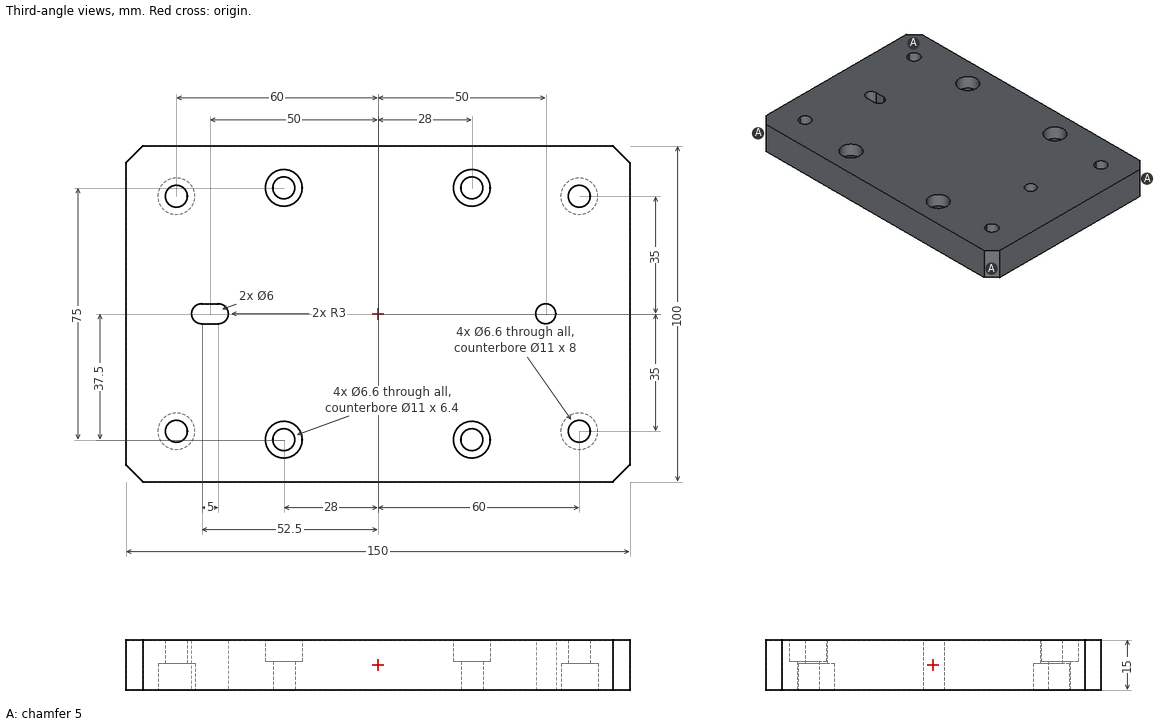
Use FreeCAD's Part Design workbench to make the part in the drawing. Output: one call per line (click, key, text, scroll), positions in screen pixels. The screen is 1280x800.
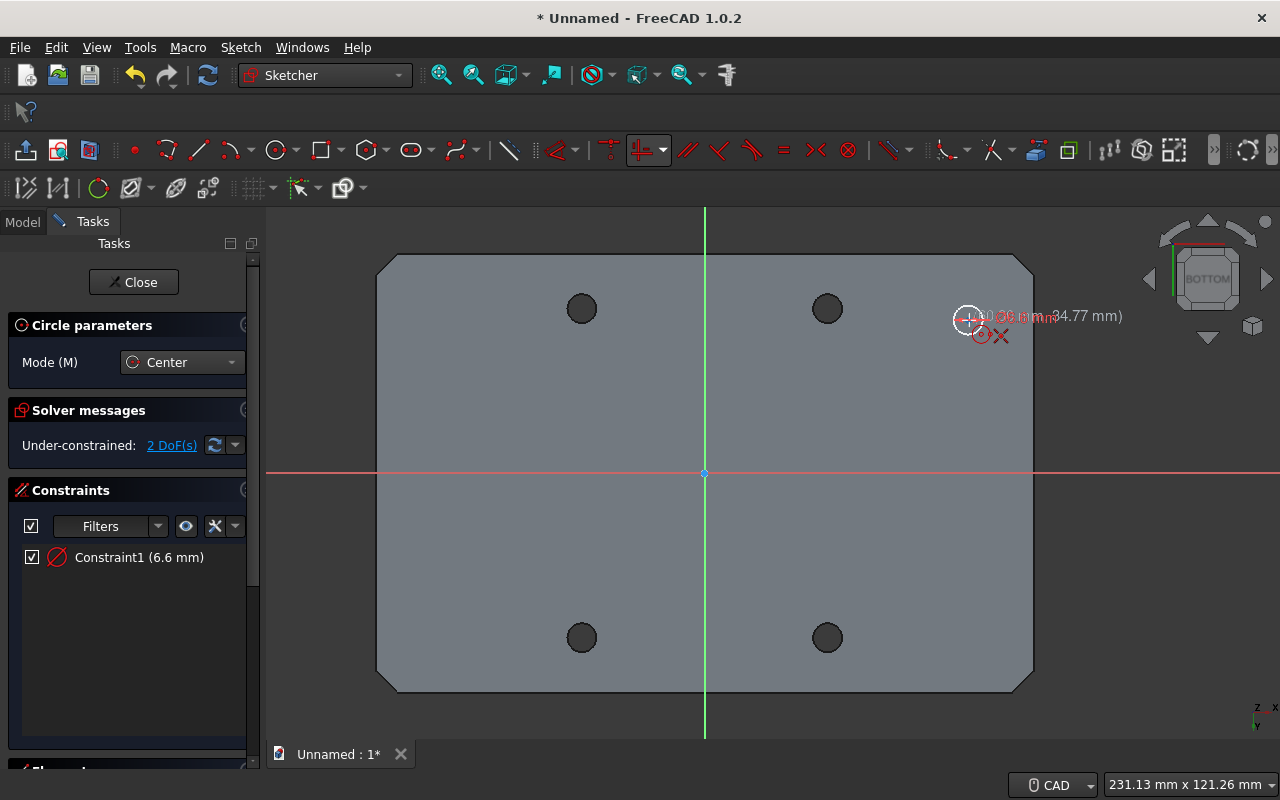
scroll(968, 627, up, 3)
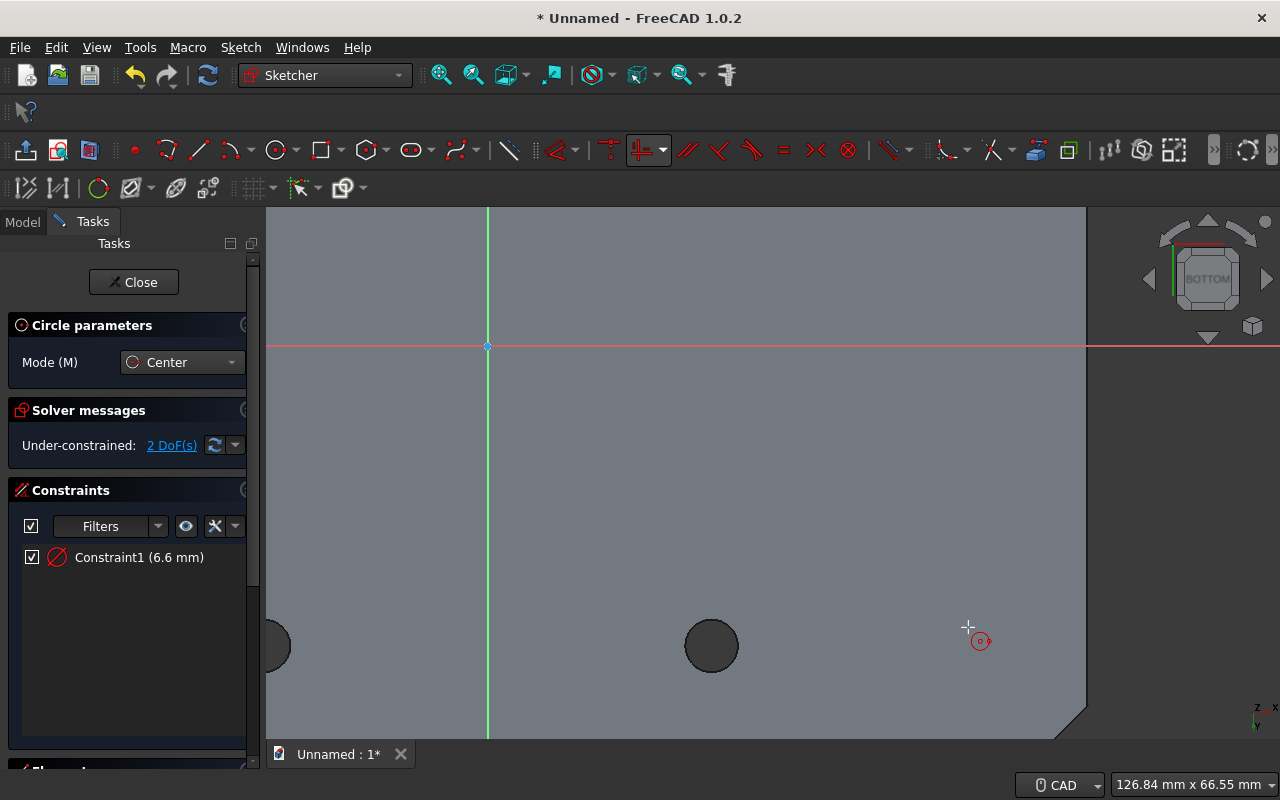
click(967, 626)
move(986, 607)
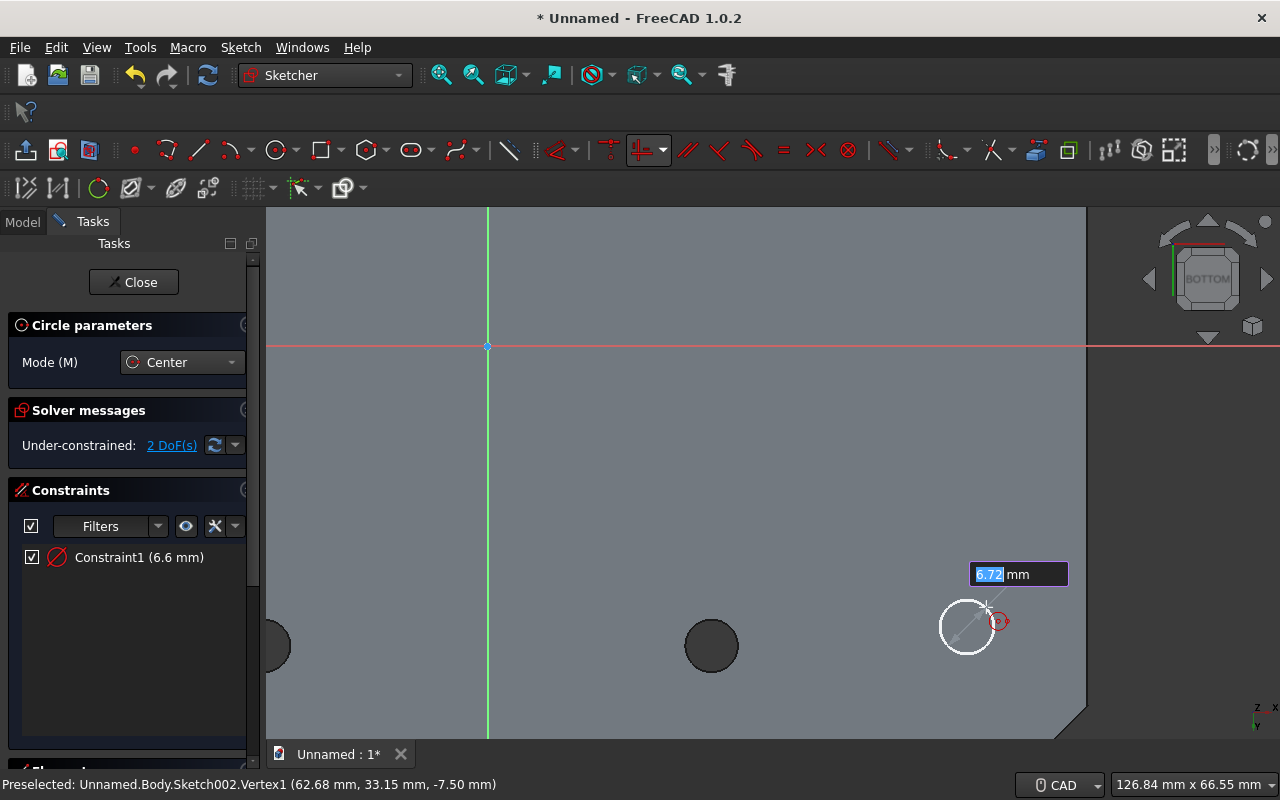
text(6.6)
key(Return)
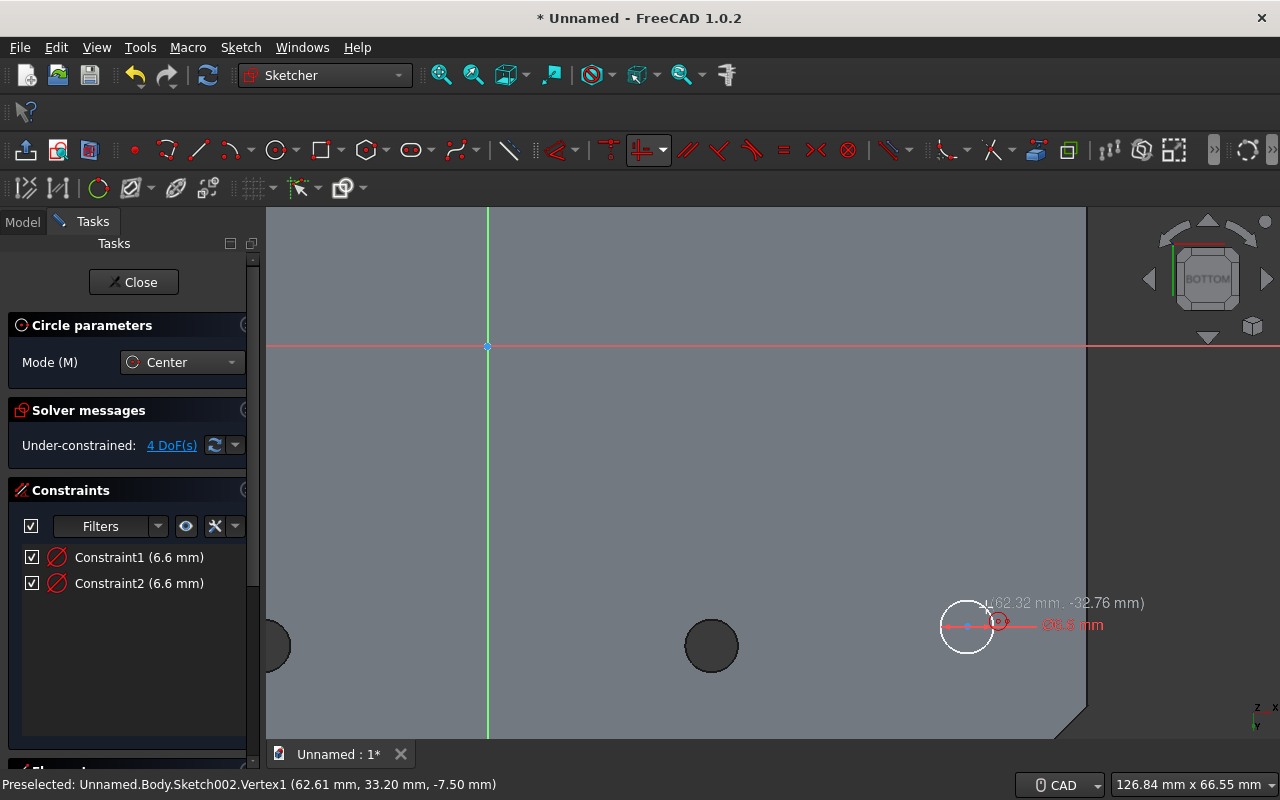
scroll(968, 627, down, 3)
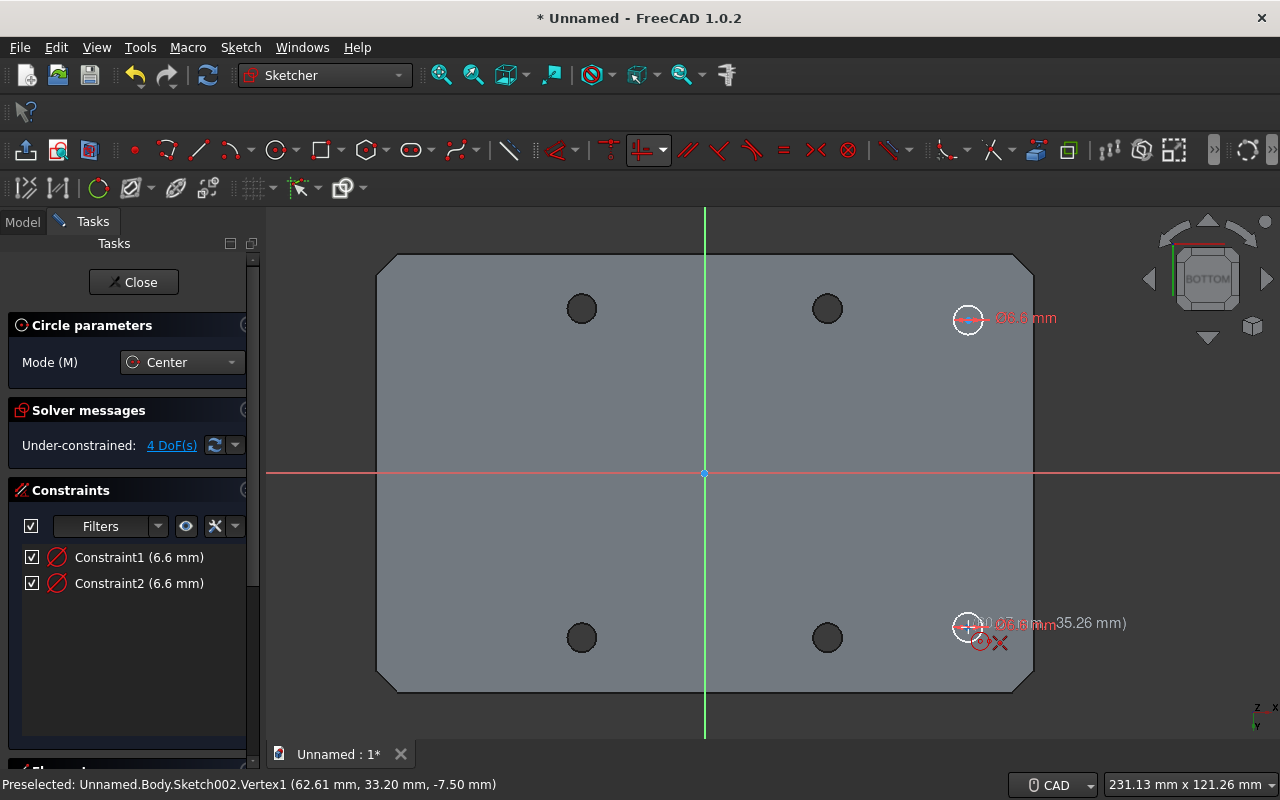
scroll(442, 627, up, 3)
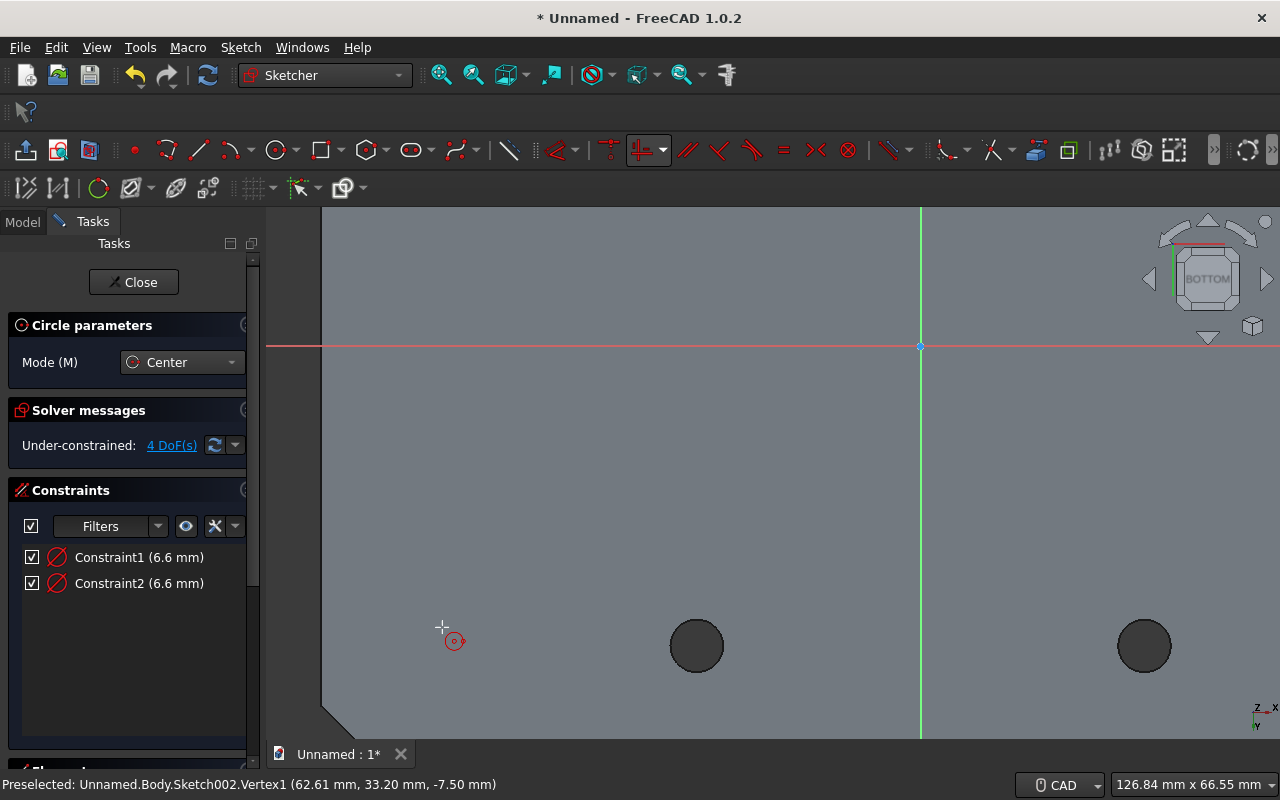
click(441, 626)
move(460, 607)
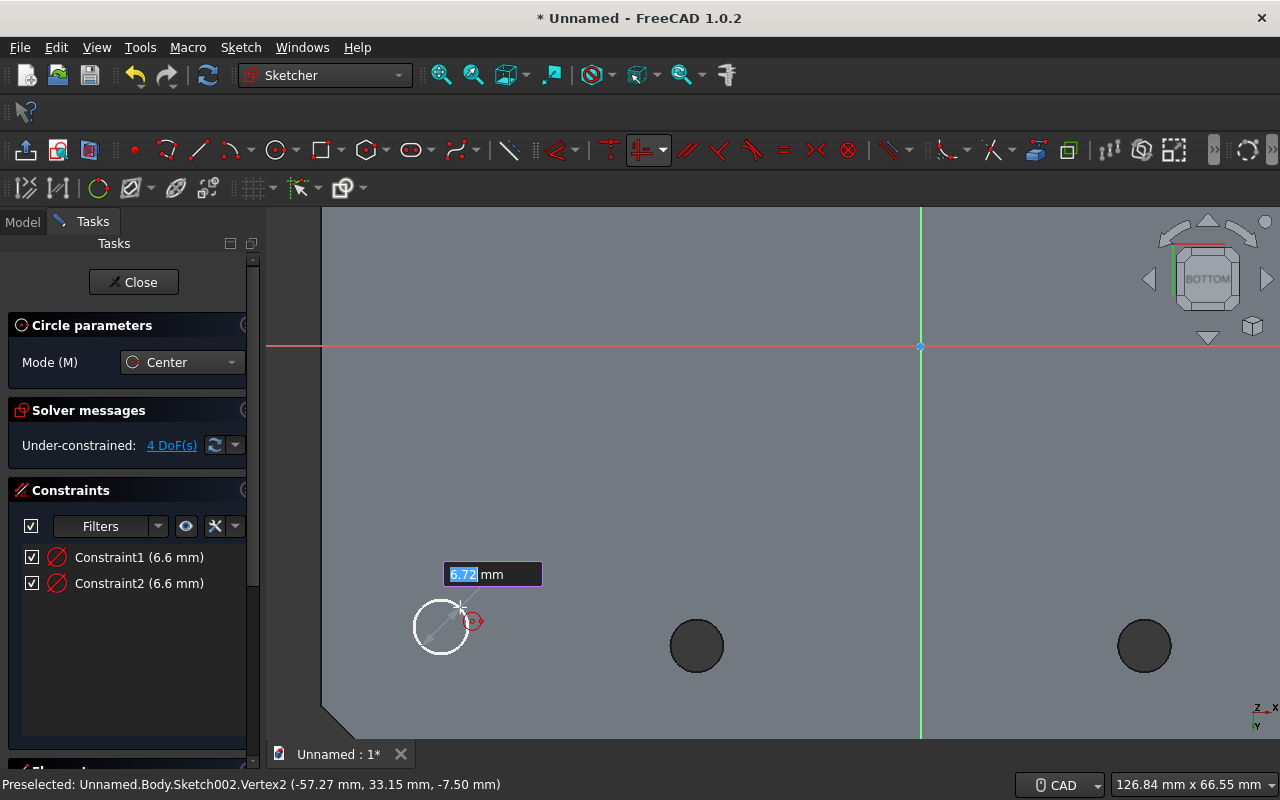
text(6.6)
key(Return)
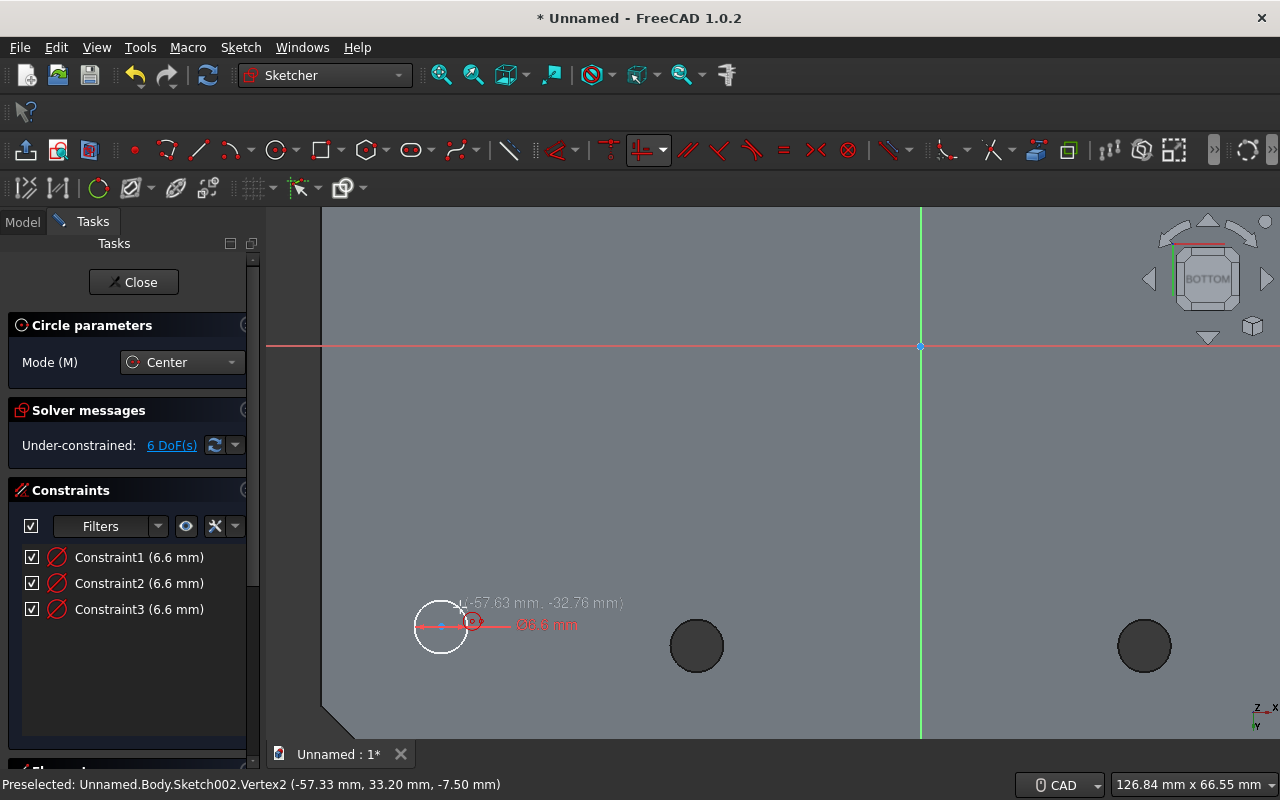
scroll(442, 627, down, 3)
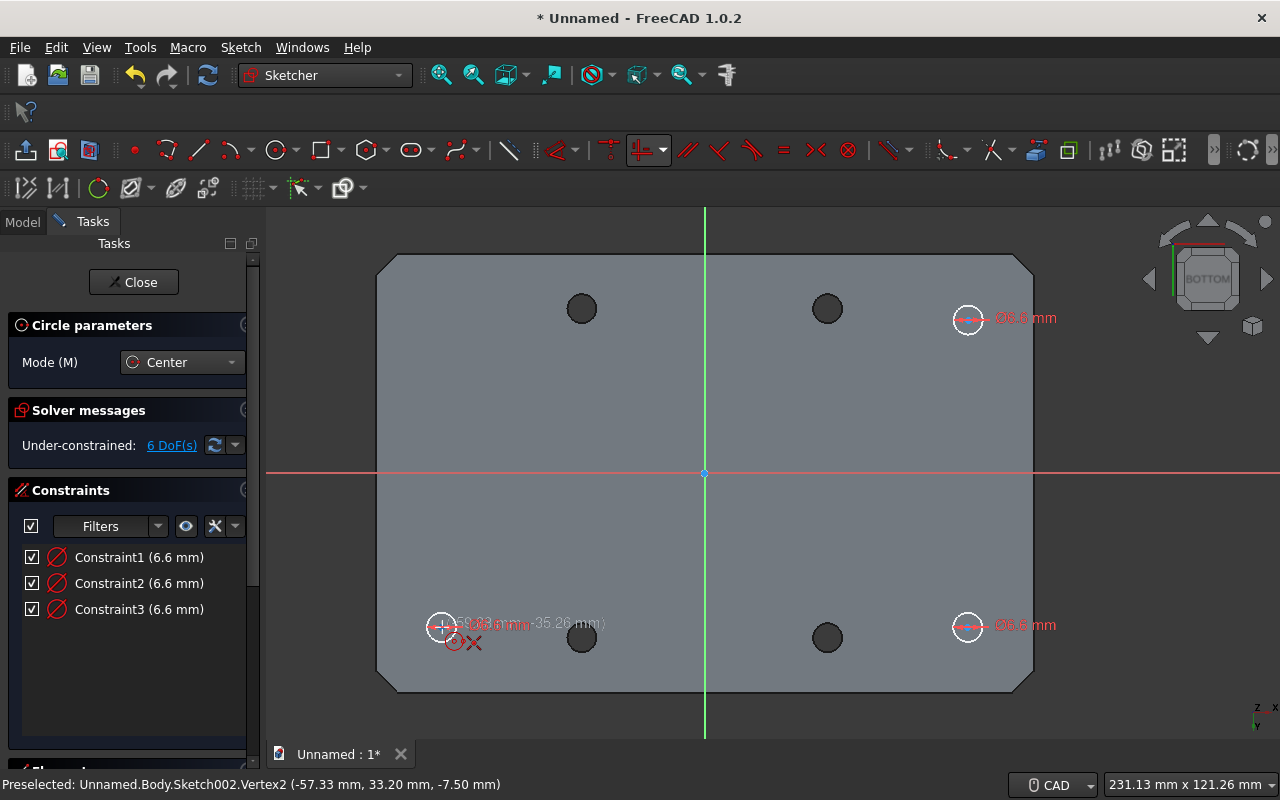
scroll(442, 320, up, 3)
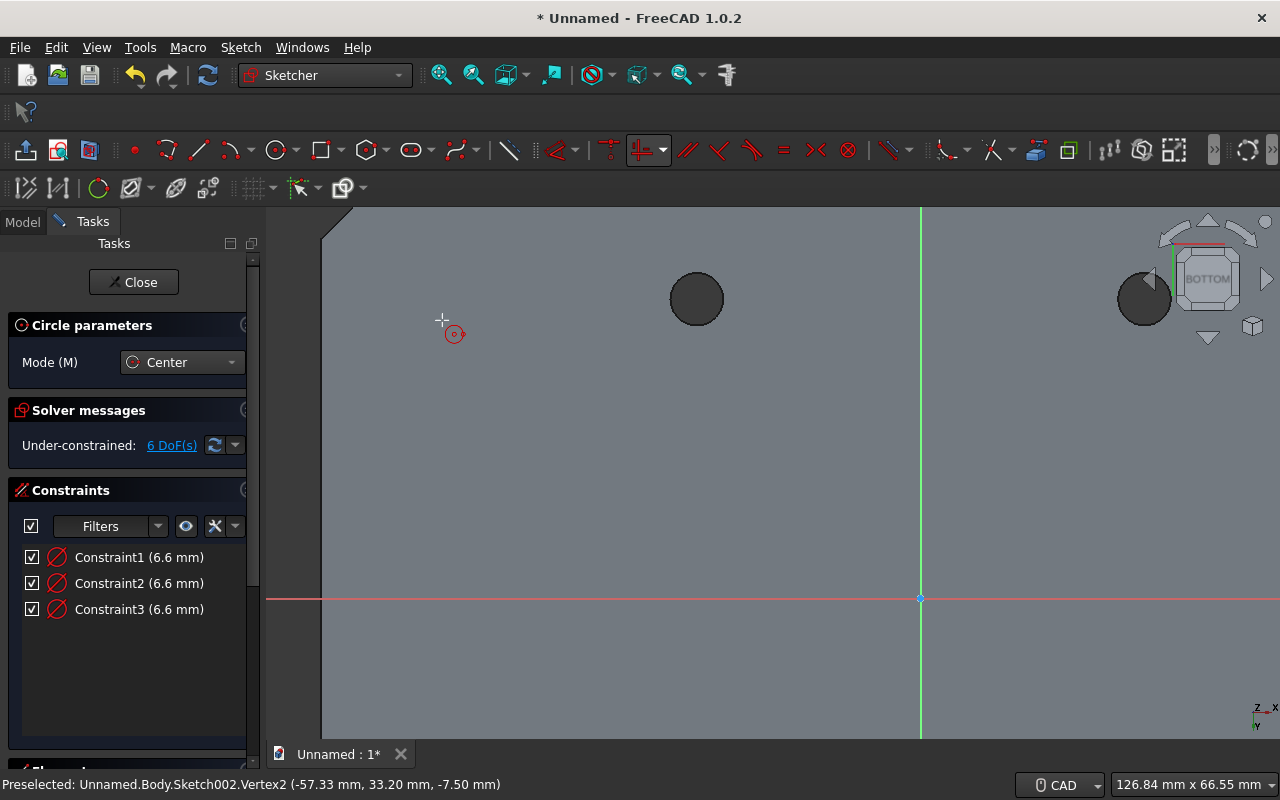
click(441, 319)
move(460, 301)